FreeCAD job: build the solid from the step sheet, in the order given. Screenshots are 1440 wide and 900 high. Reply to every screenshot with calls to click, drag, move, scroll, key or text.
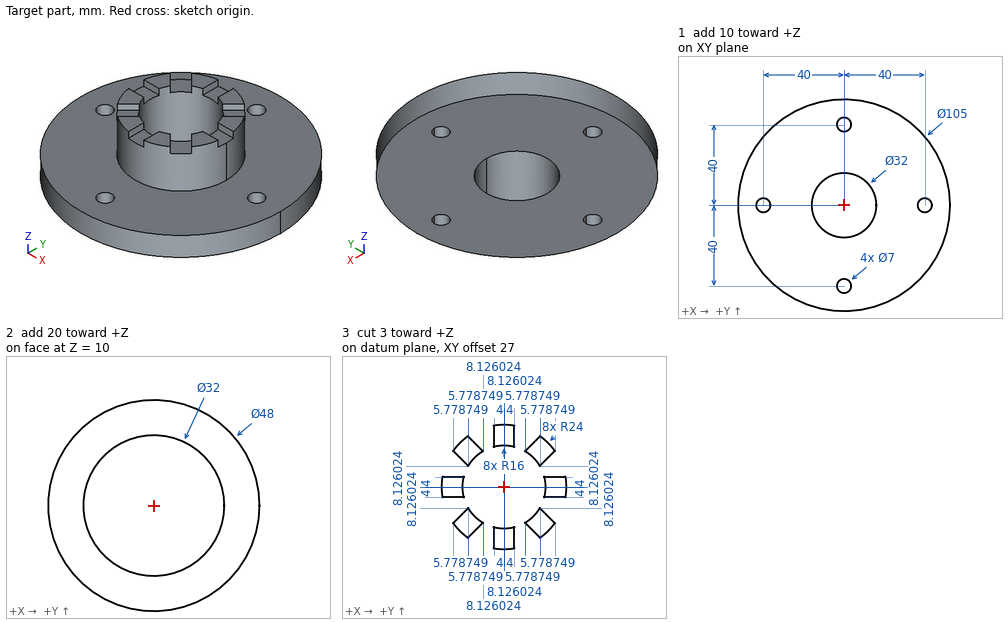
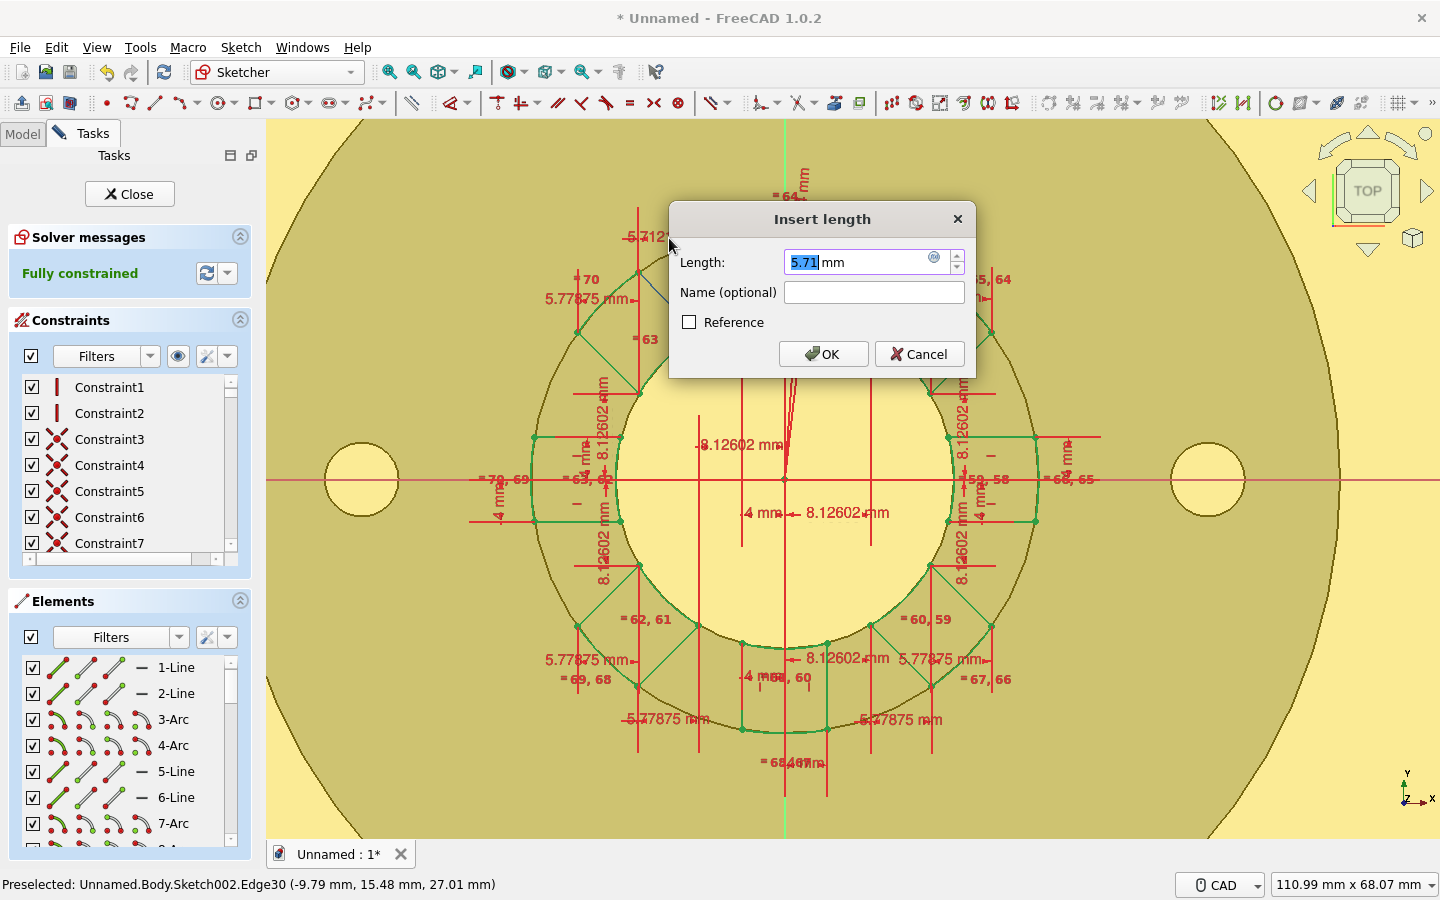
text(5.778749)
key(Return)
key(Escape)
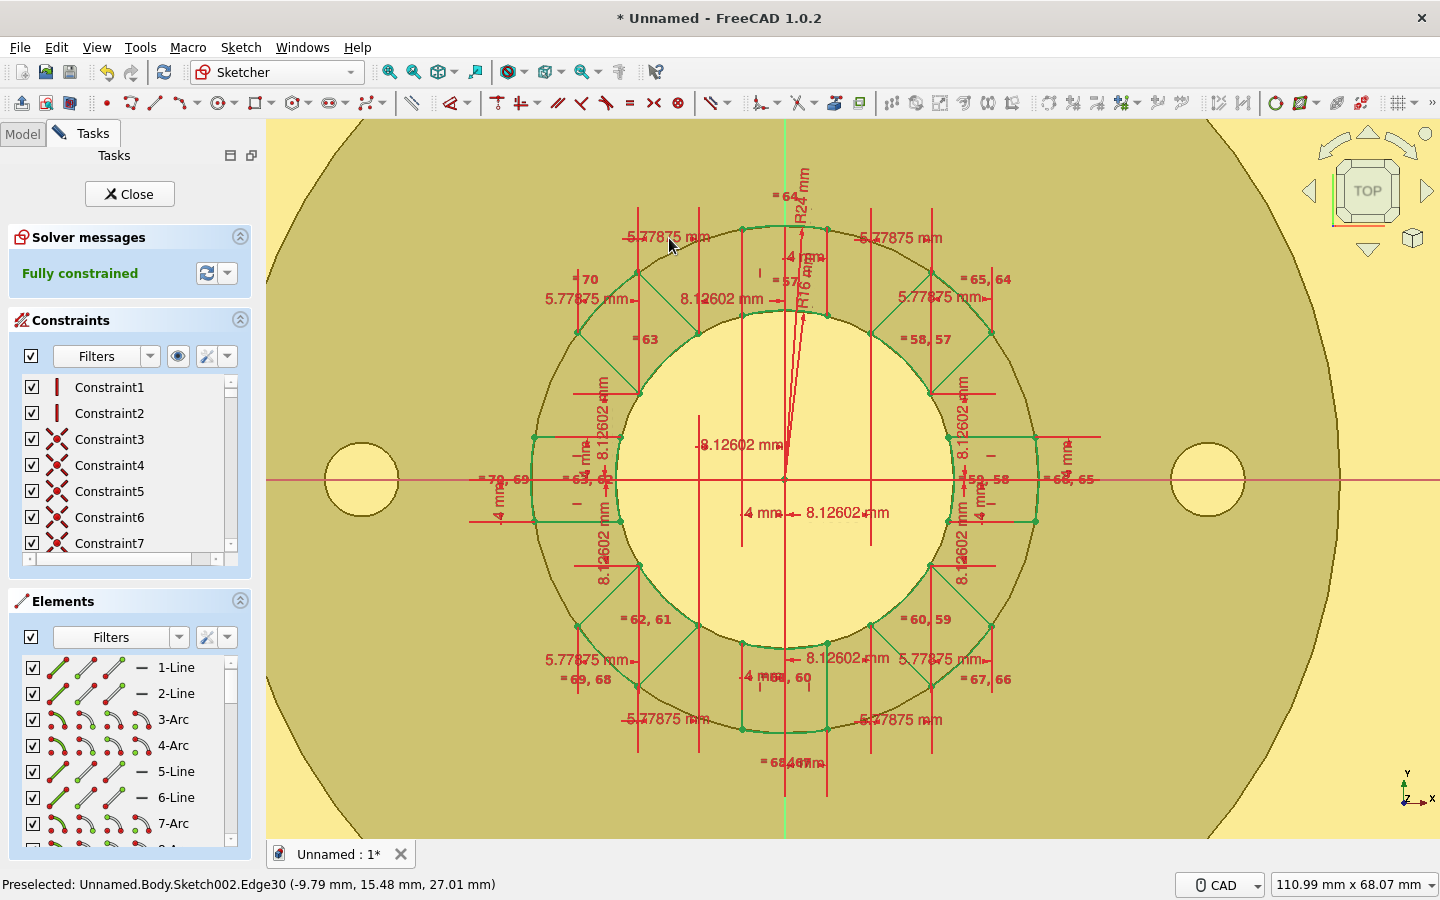
click(130, 194)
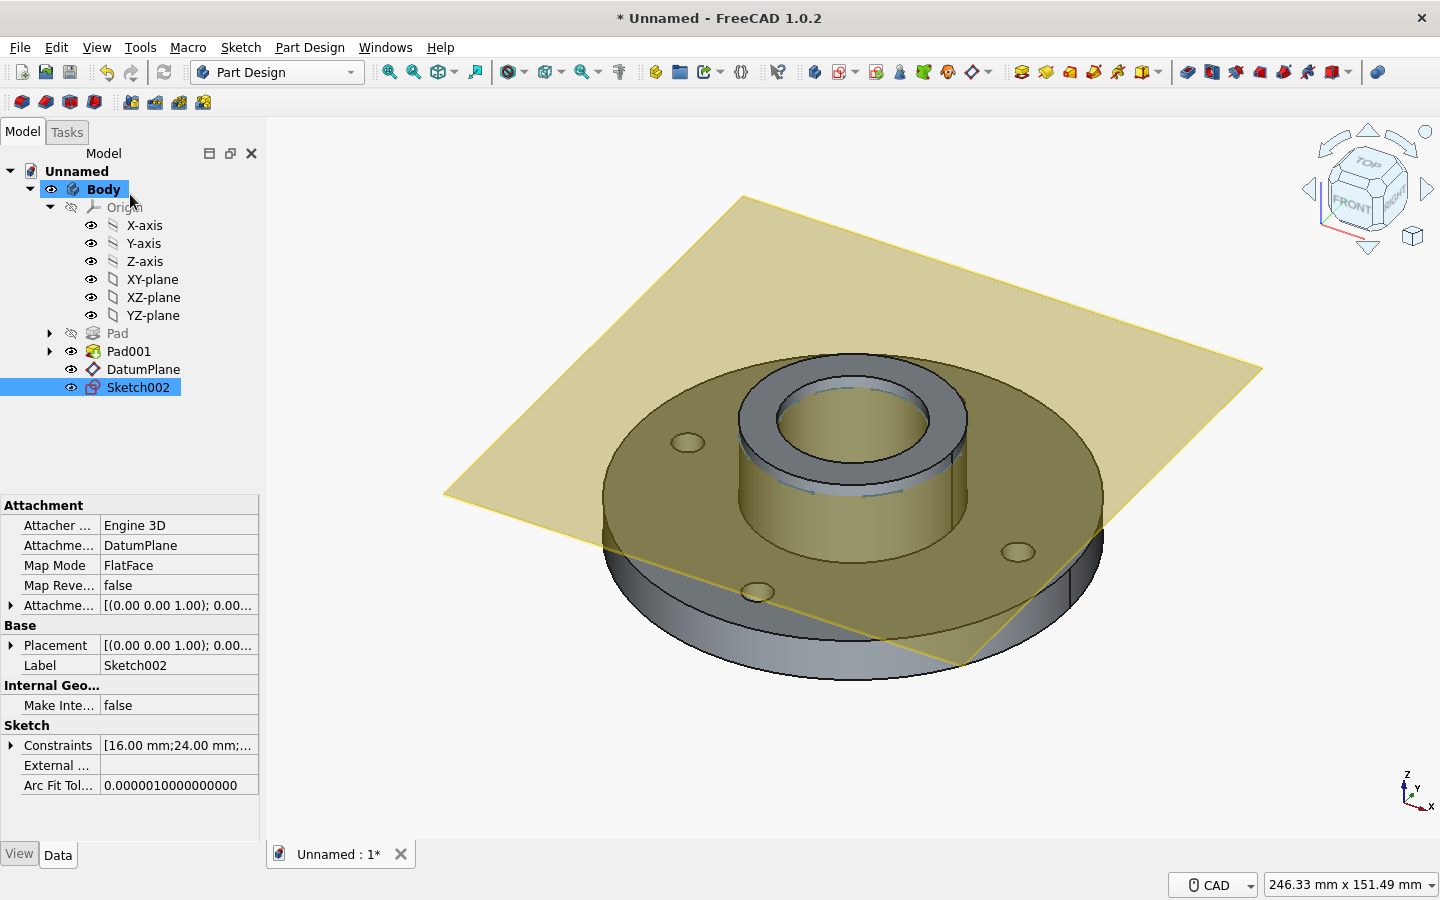
click(1188, 72)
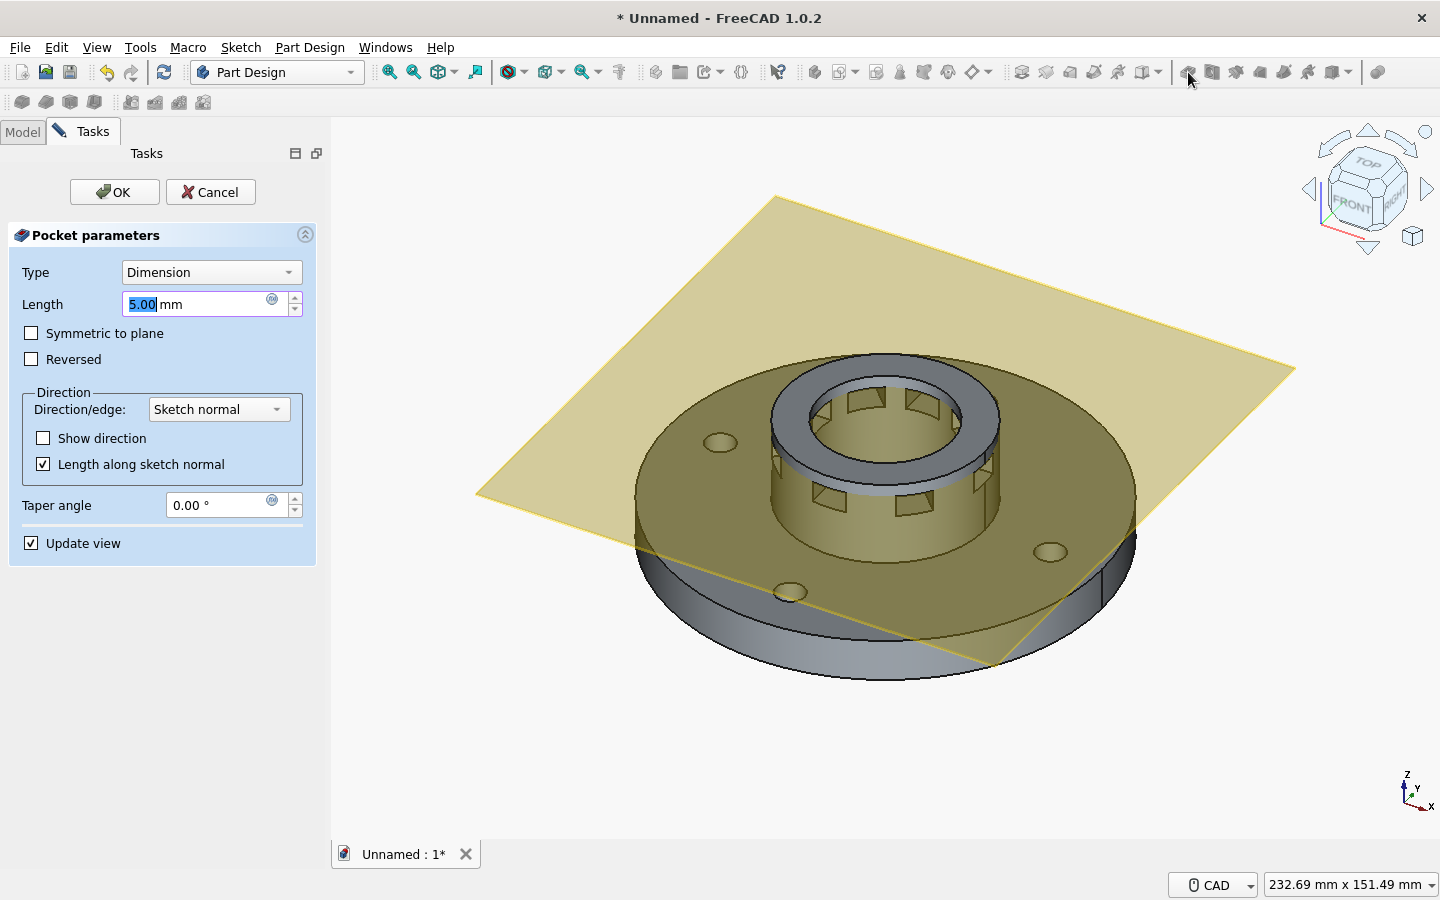
text(3)
key(Tab)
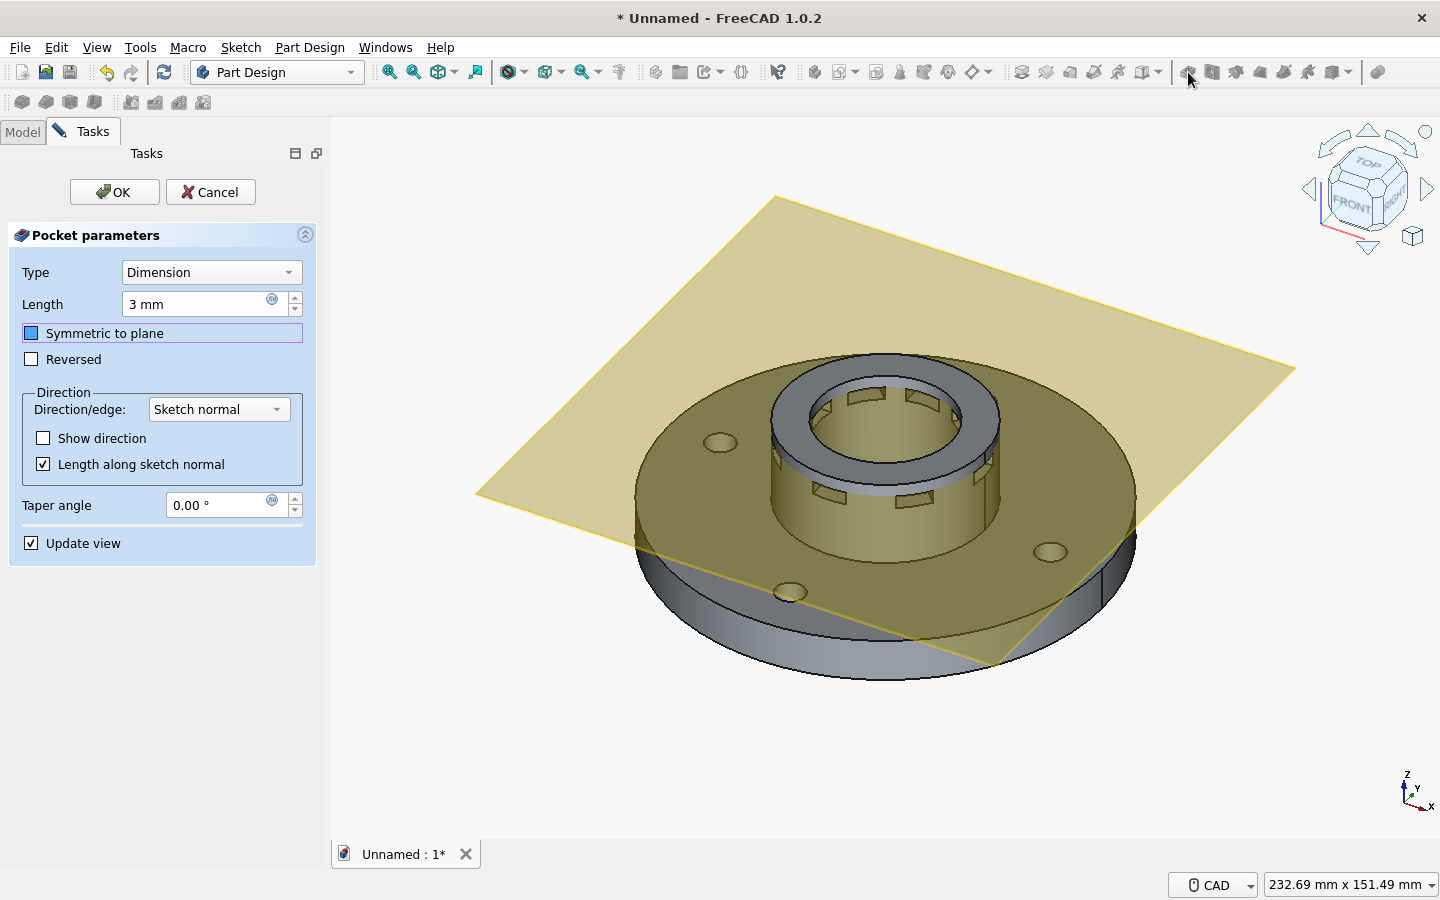
click(30, 359)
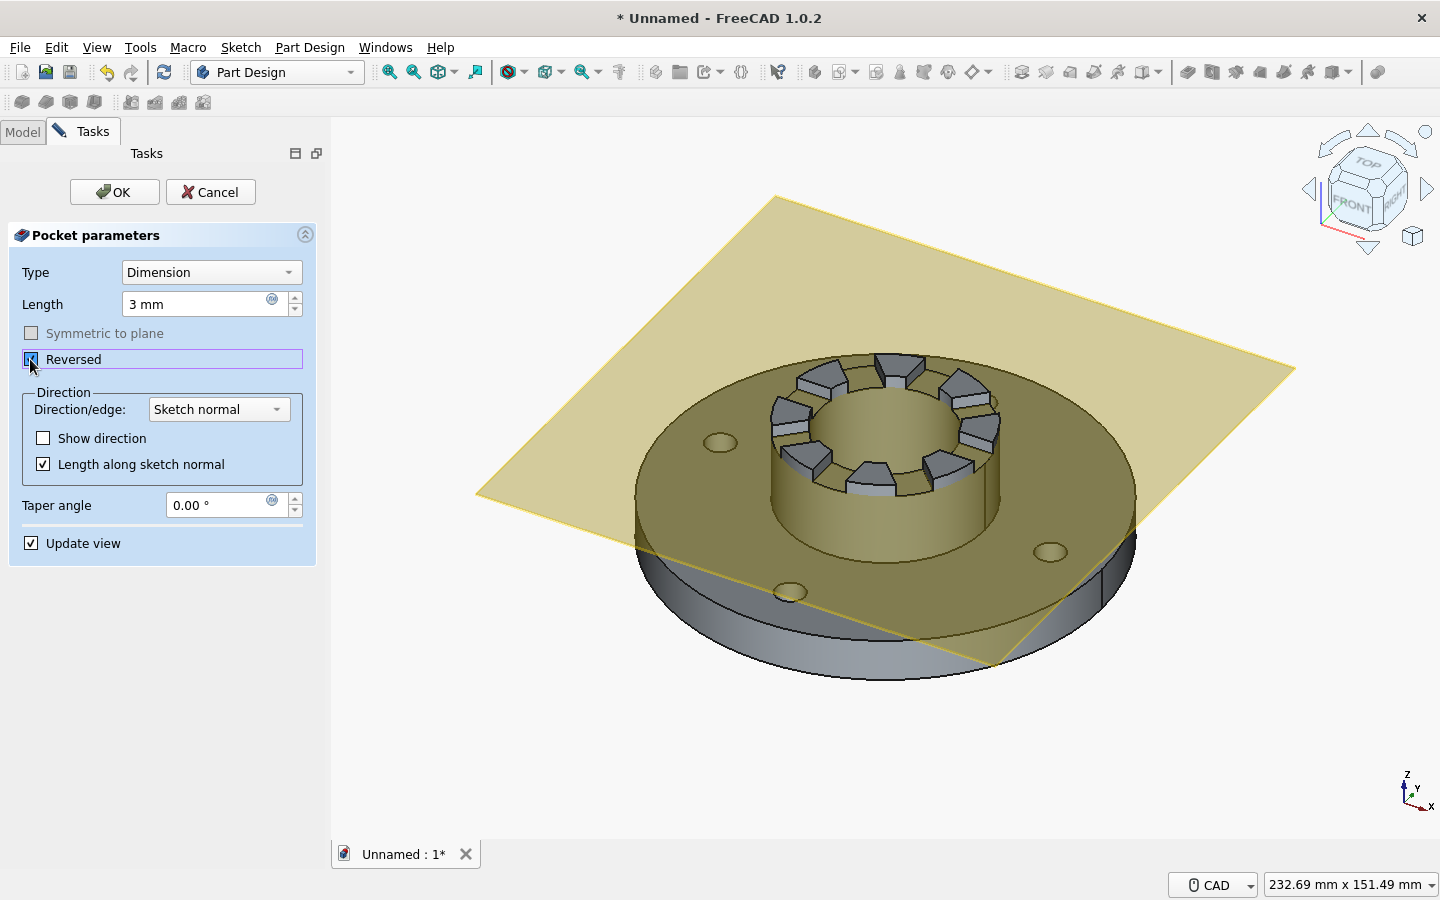
click(115, 192)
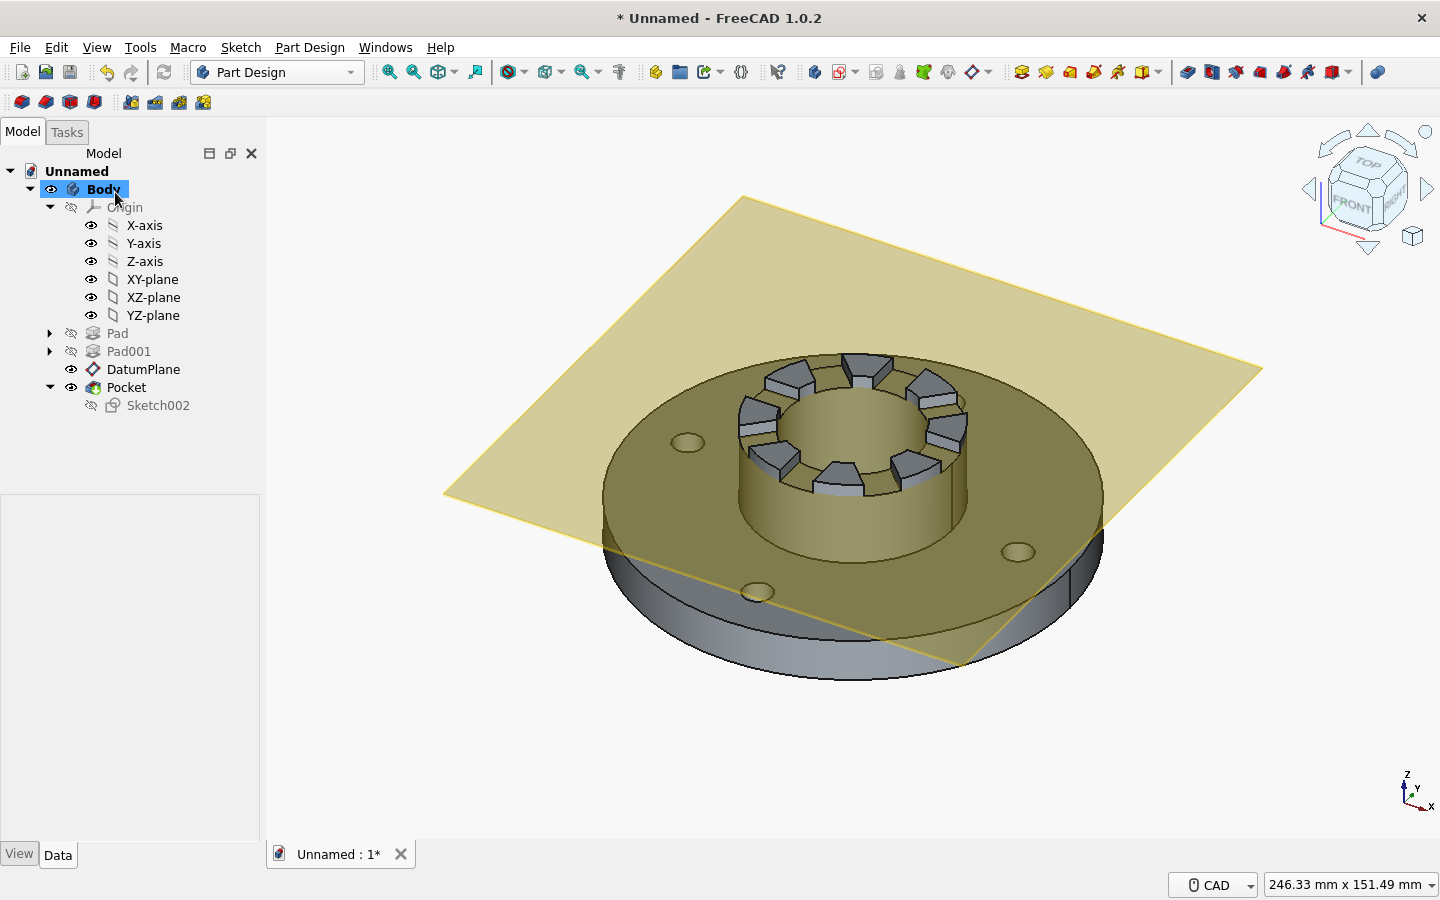
click(116, 369)
key(space)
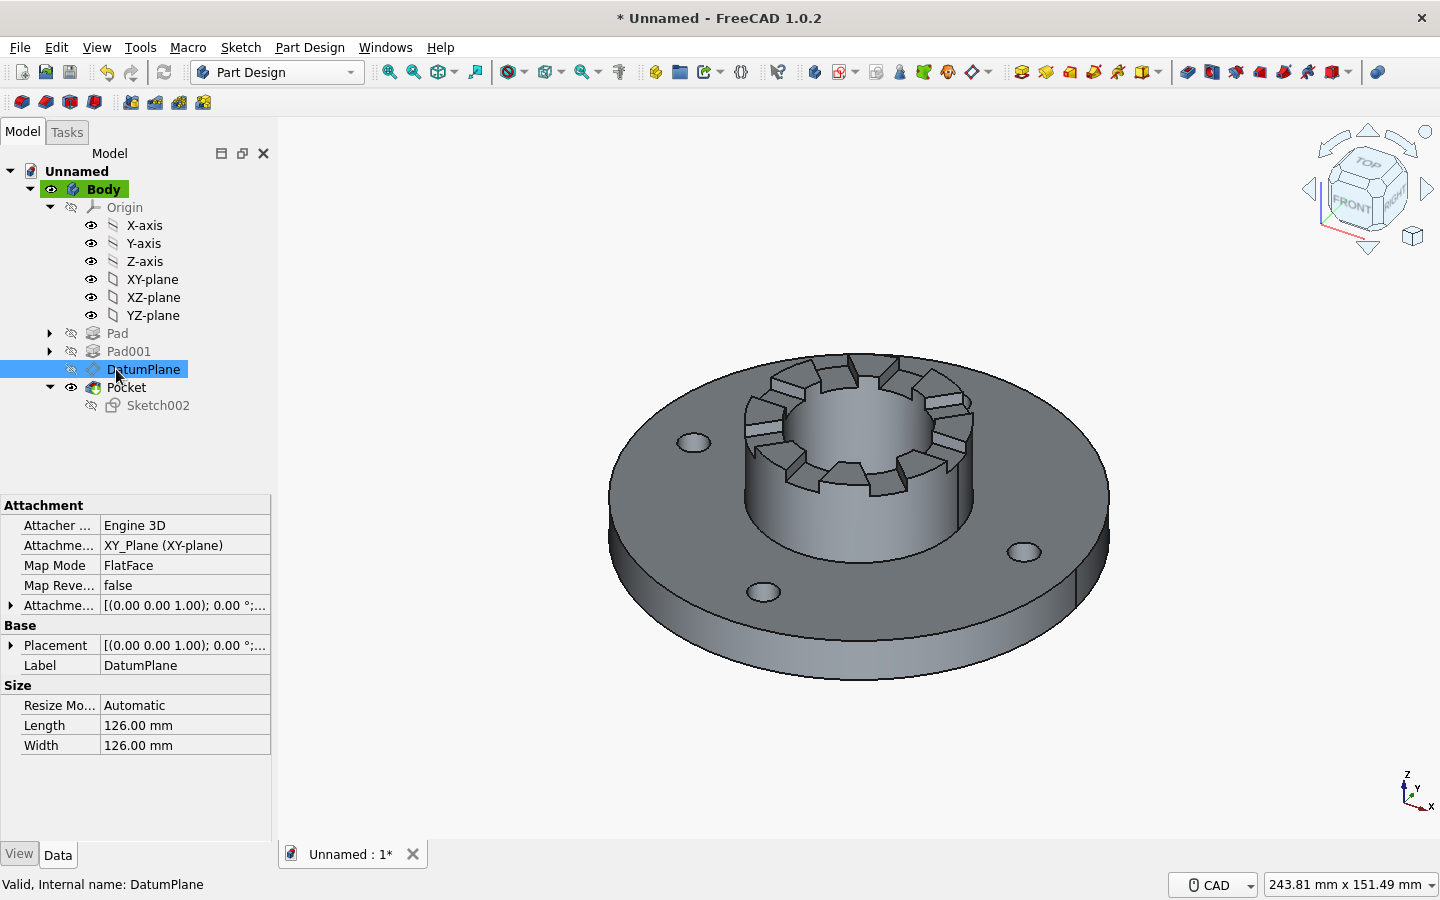
key(0)